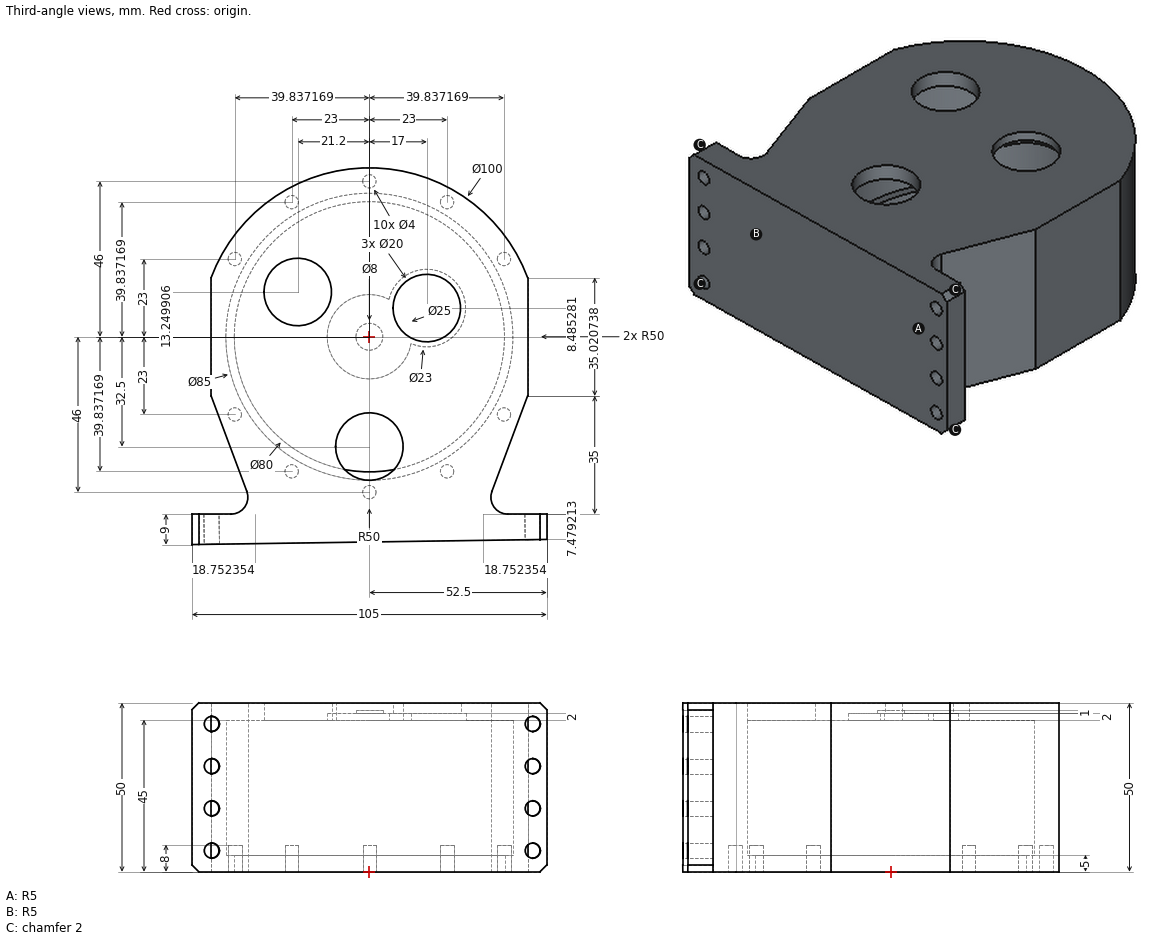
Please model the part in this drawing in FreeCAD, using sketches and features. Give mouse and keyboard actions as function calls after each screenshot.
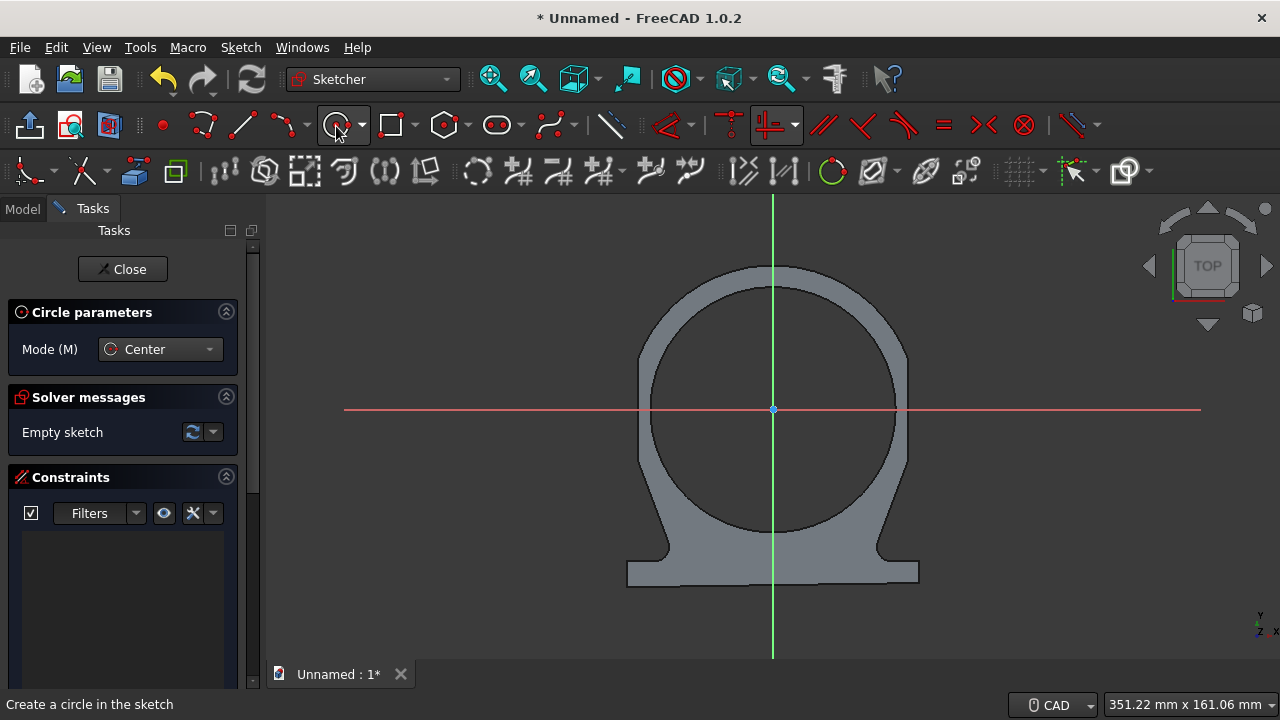
click(773, 410)
click(860, 323)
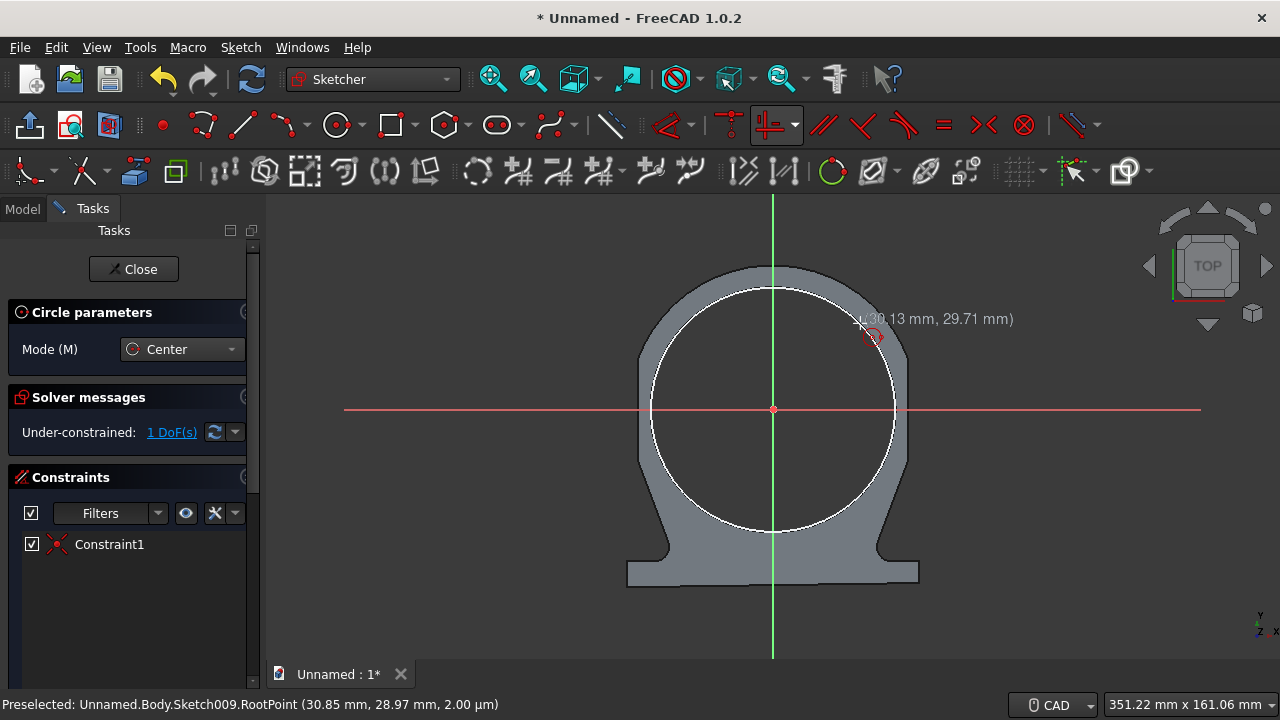
click(773, 410)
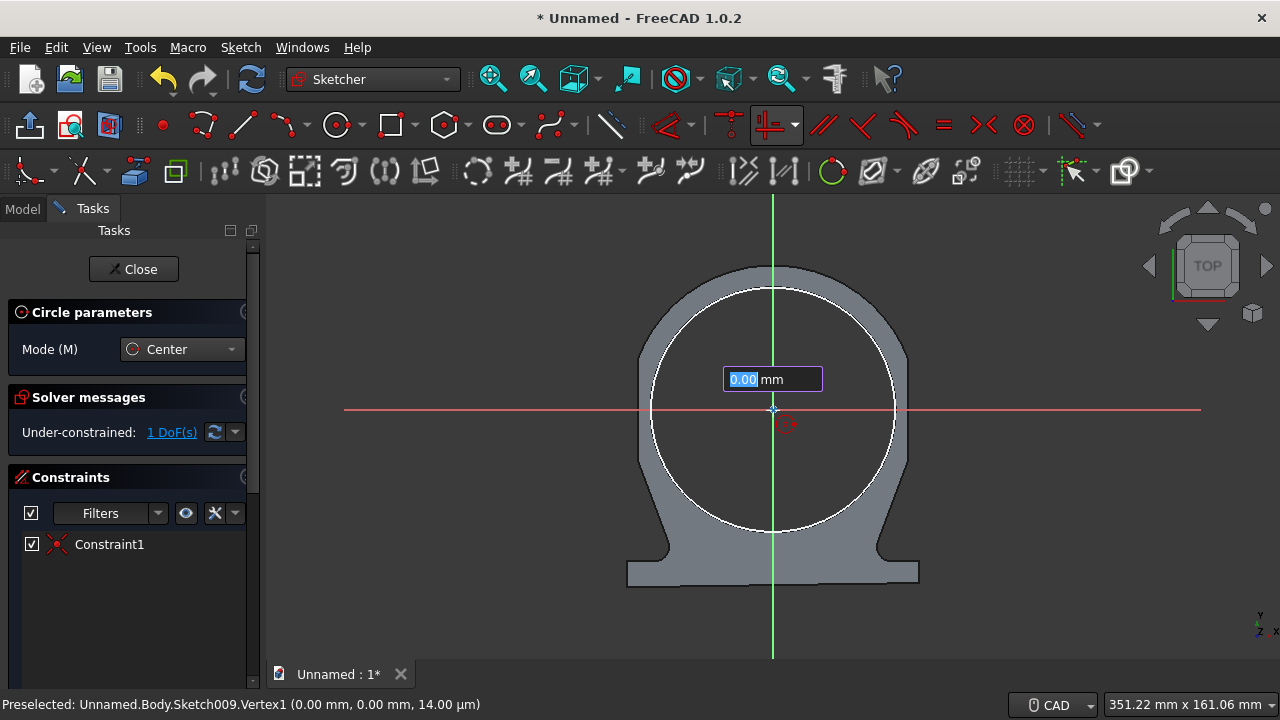
scroll(855, 328, up, 4)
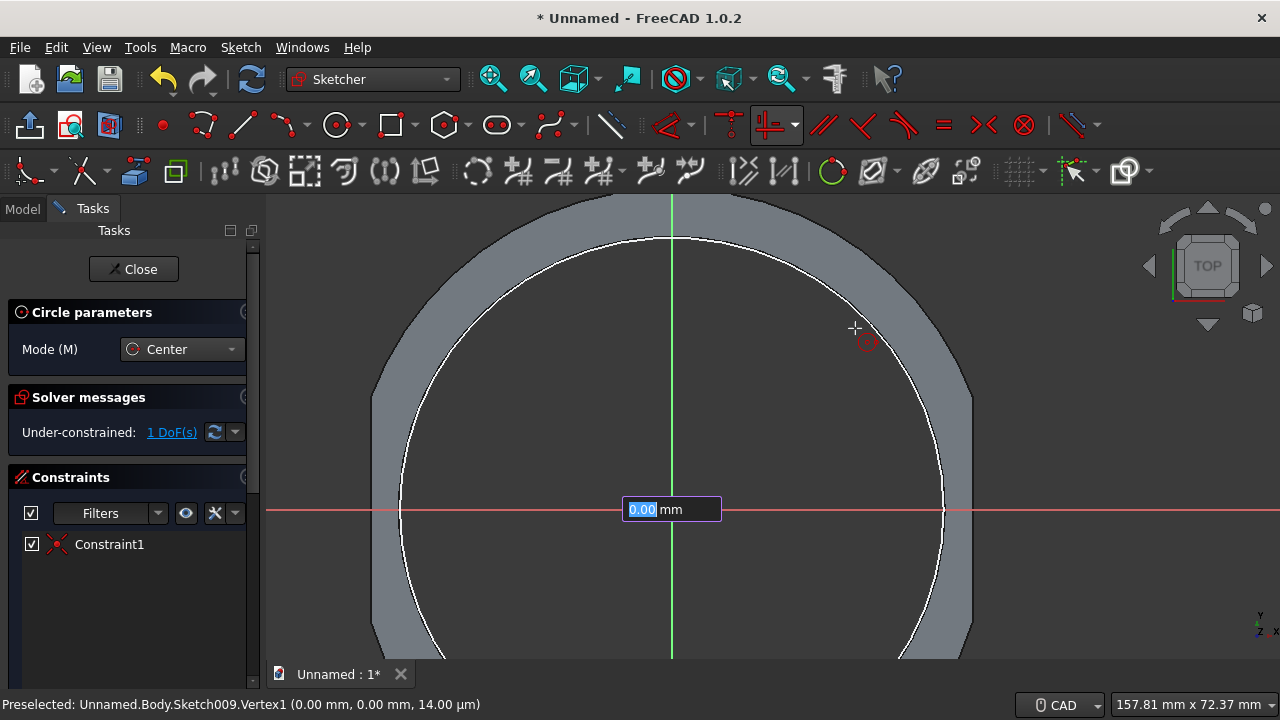
click(854, 328)
key(Escape)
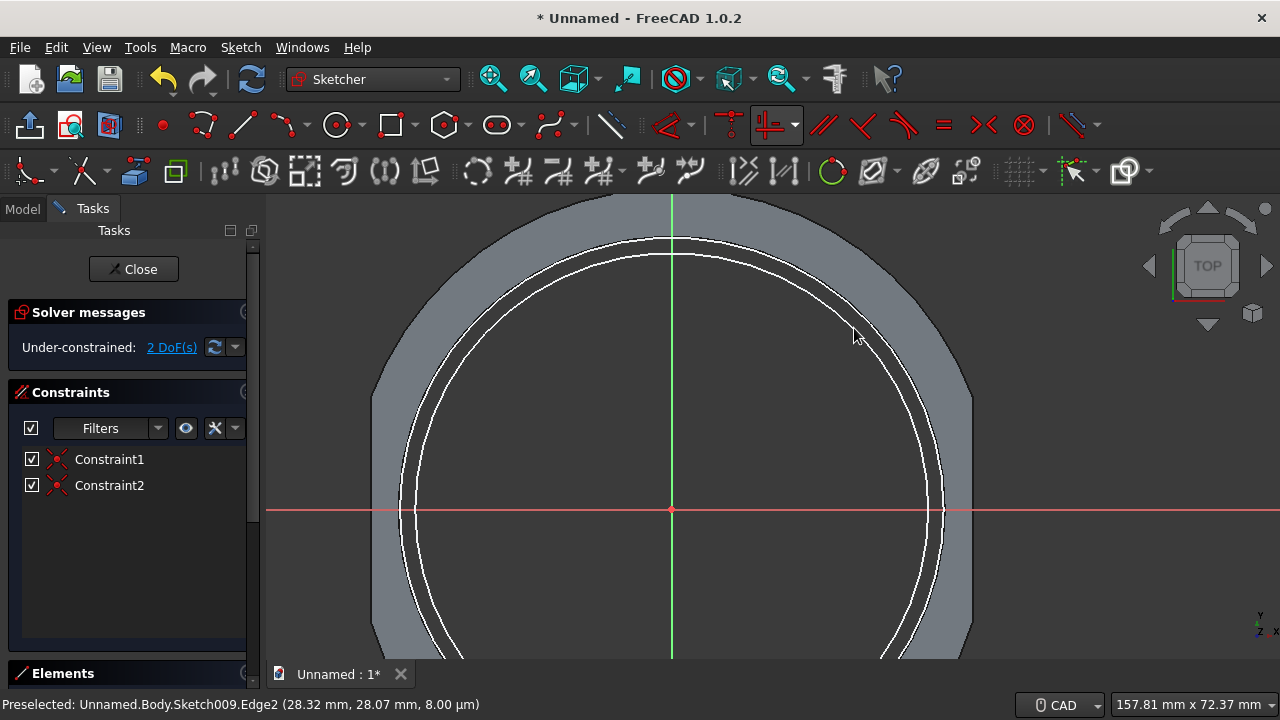
click(666, 126)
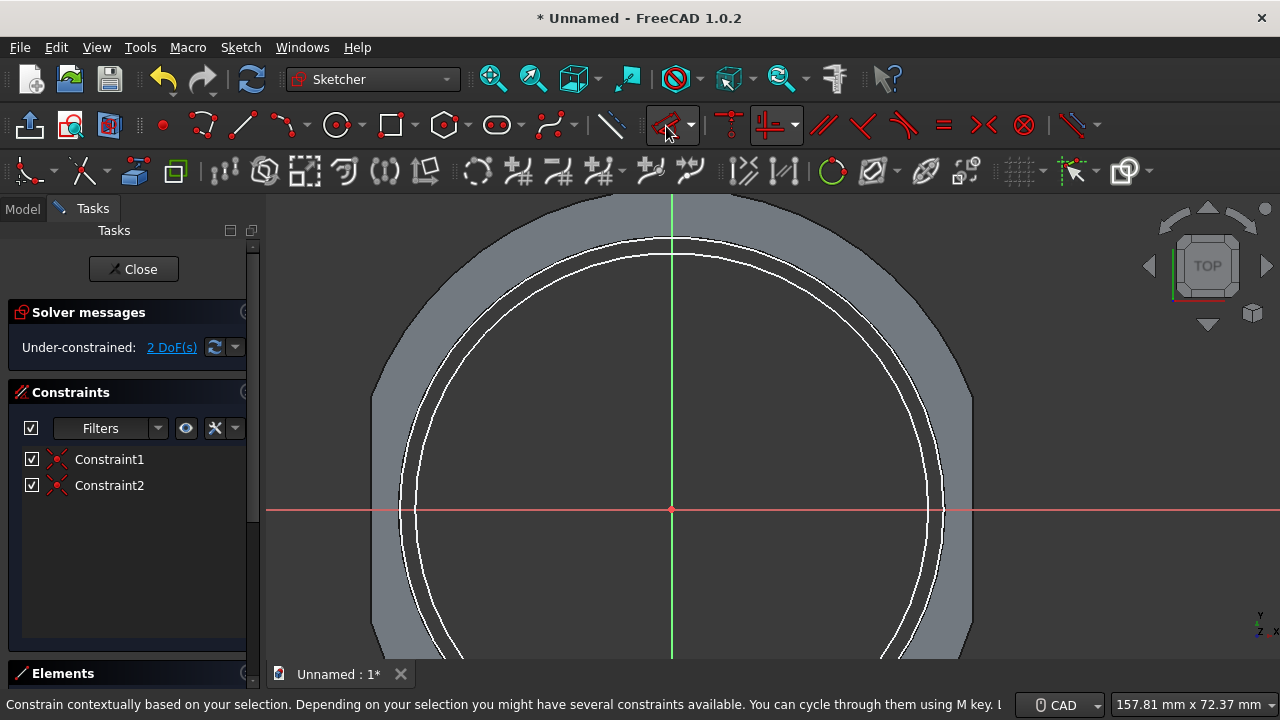
click(863, 317)
click(886, 294)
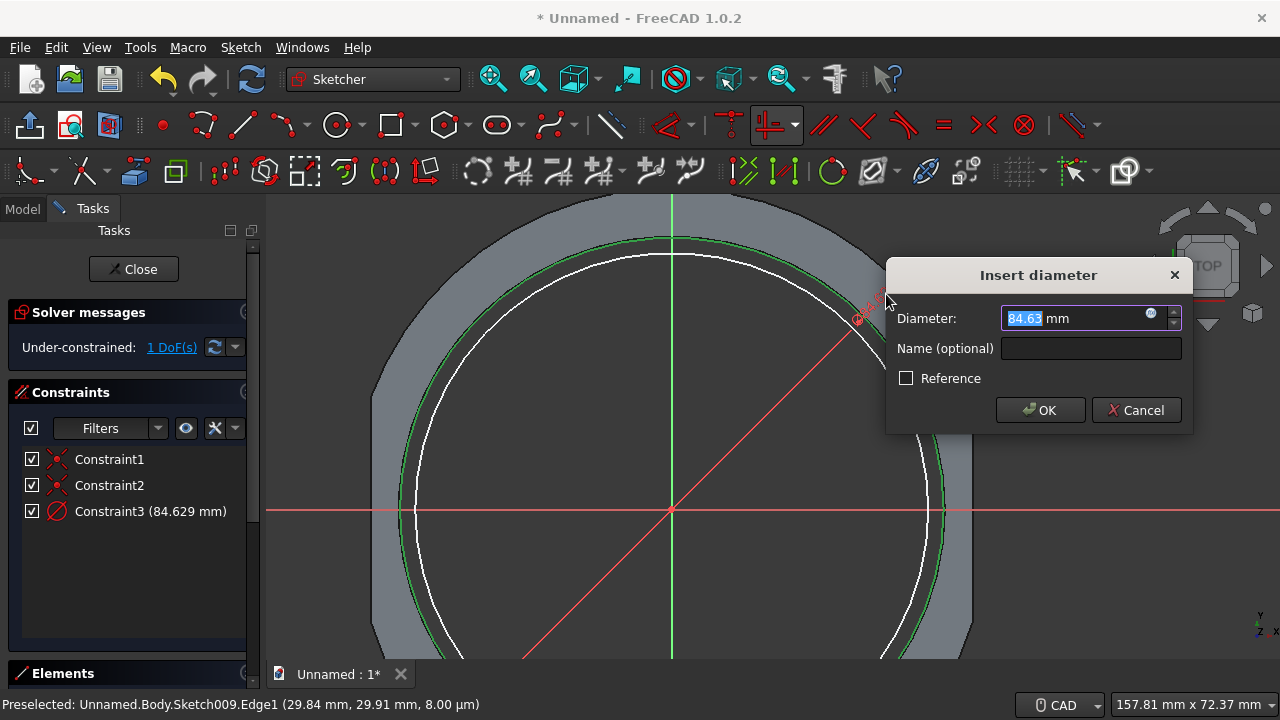
text(85)
key(Return)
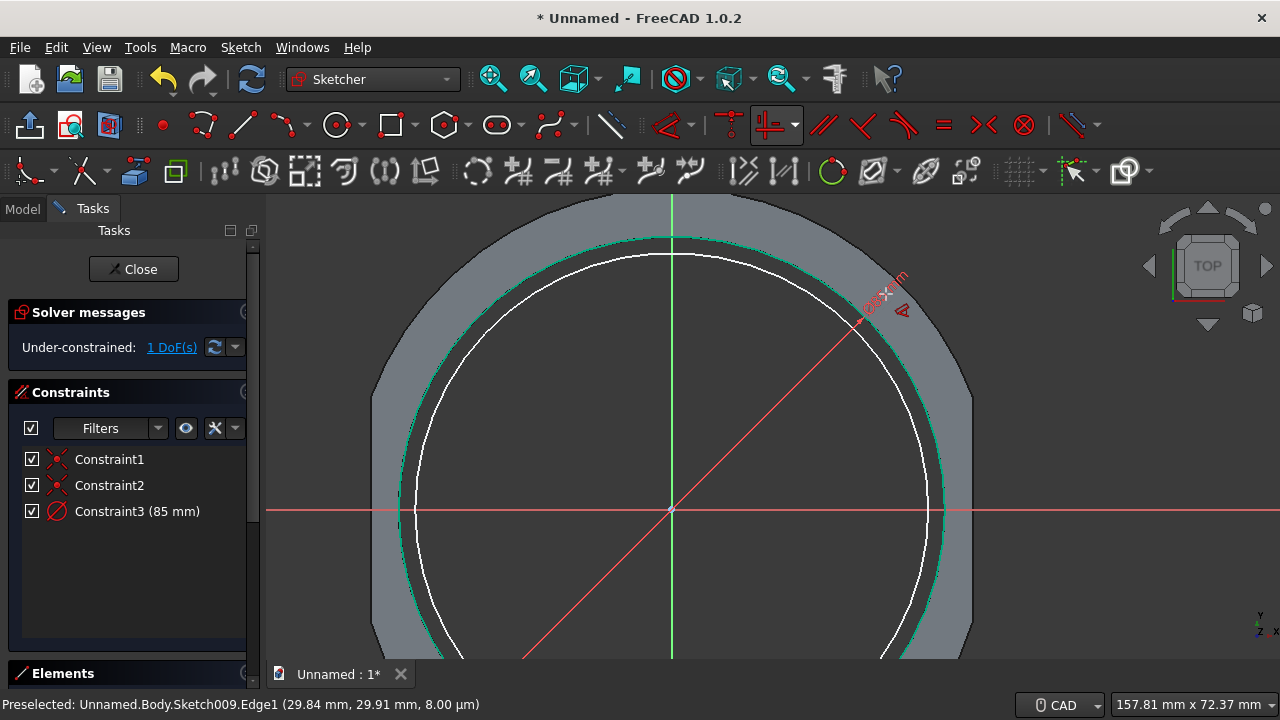
click(853, 328)
click(949, 428)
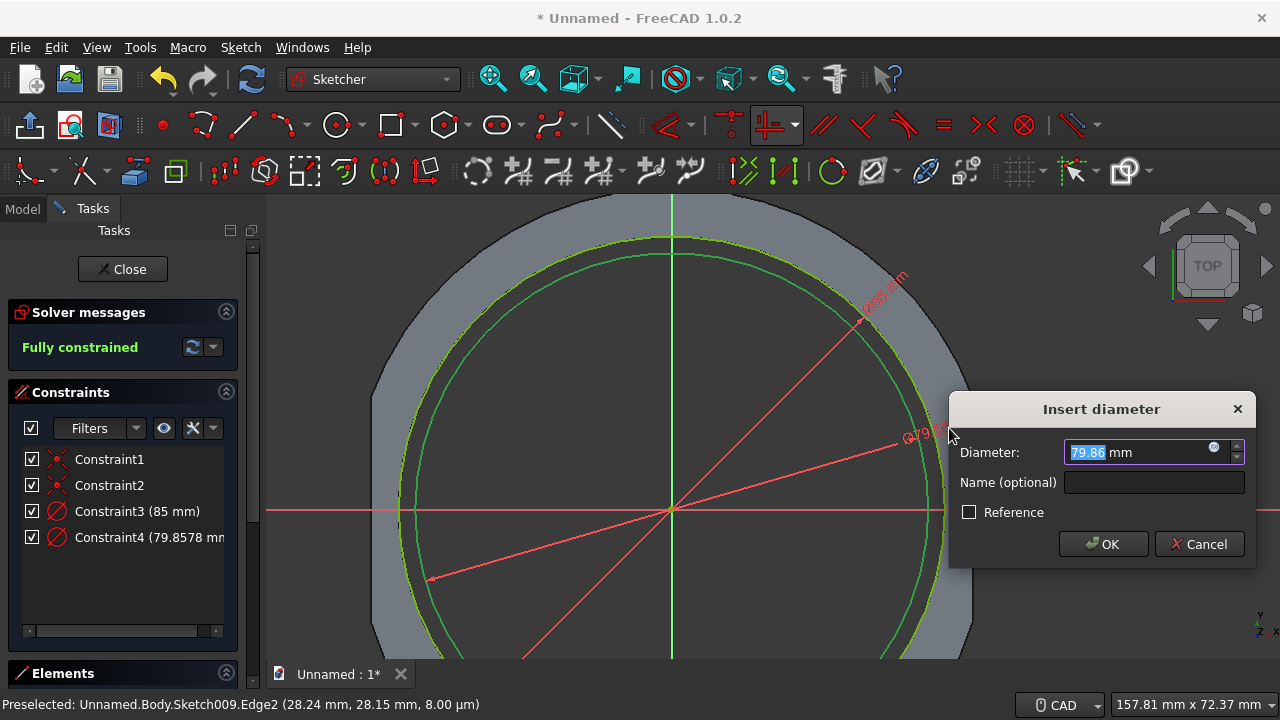
text(80)
key(Return)
key(Escape)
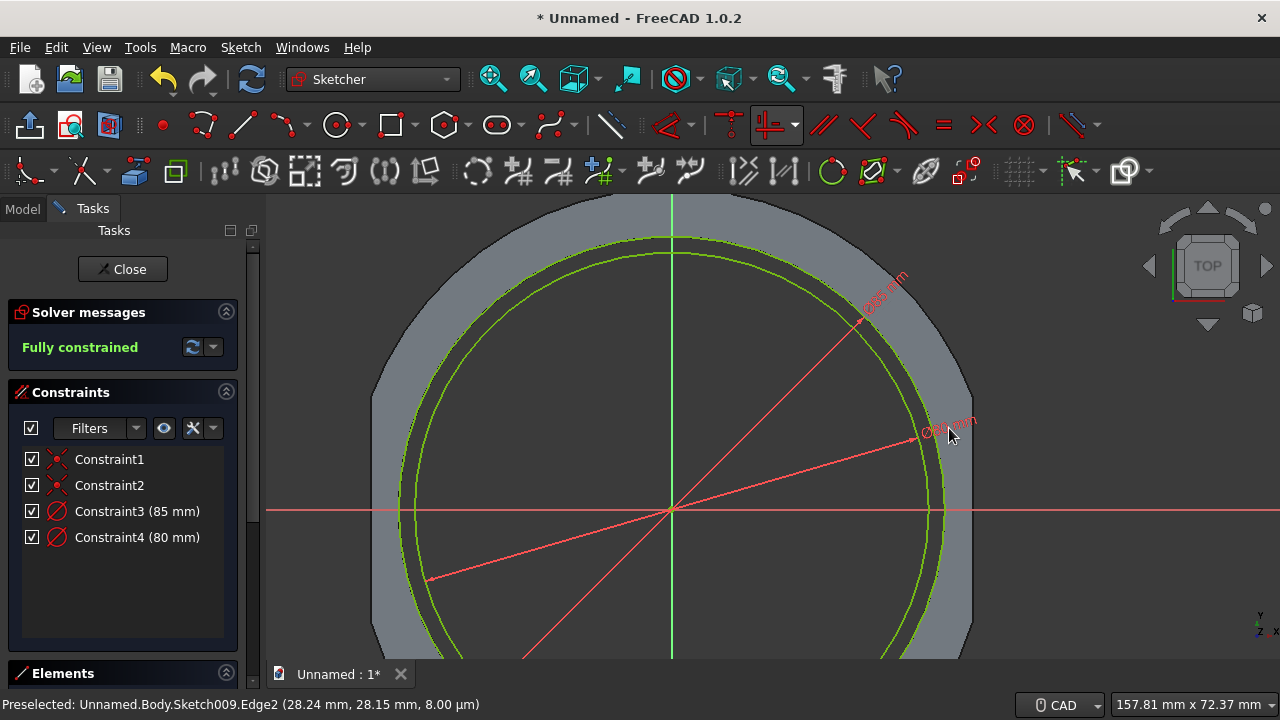
click(123, 269)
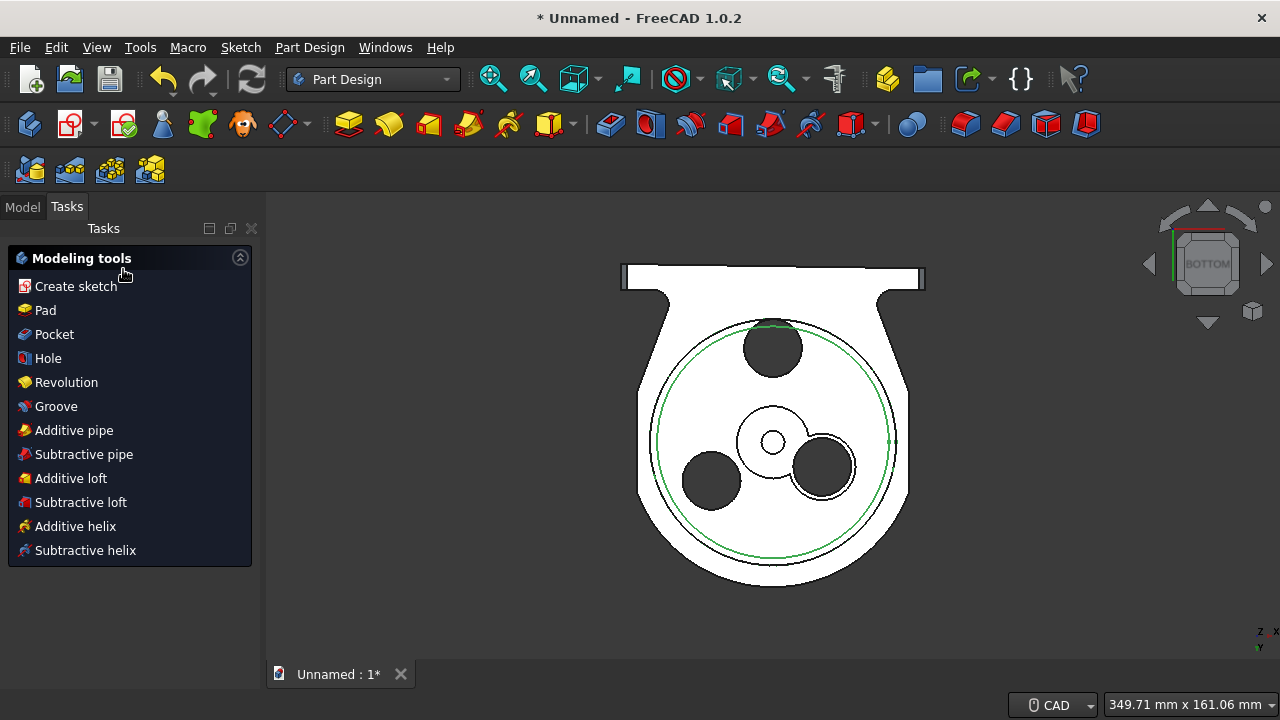
click(350, 124)